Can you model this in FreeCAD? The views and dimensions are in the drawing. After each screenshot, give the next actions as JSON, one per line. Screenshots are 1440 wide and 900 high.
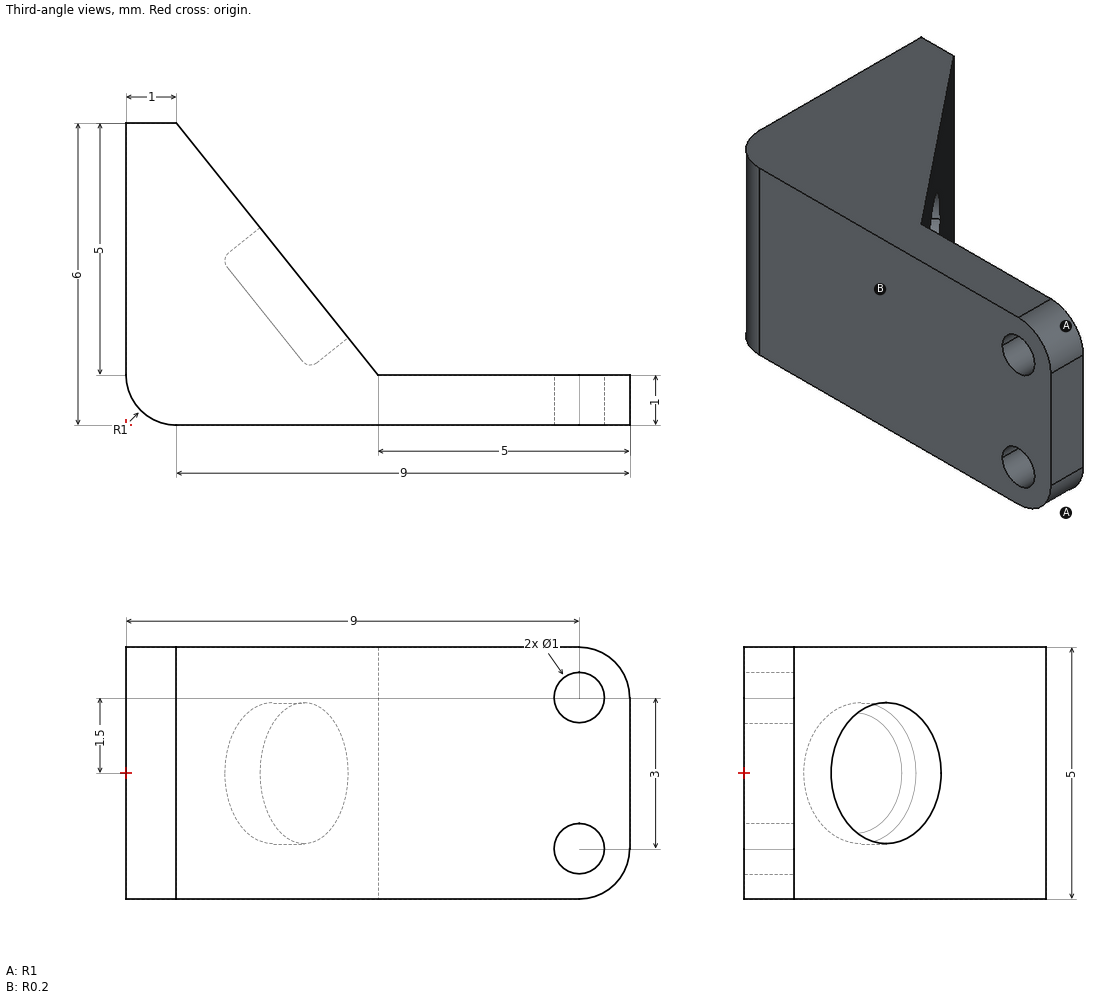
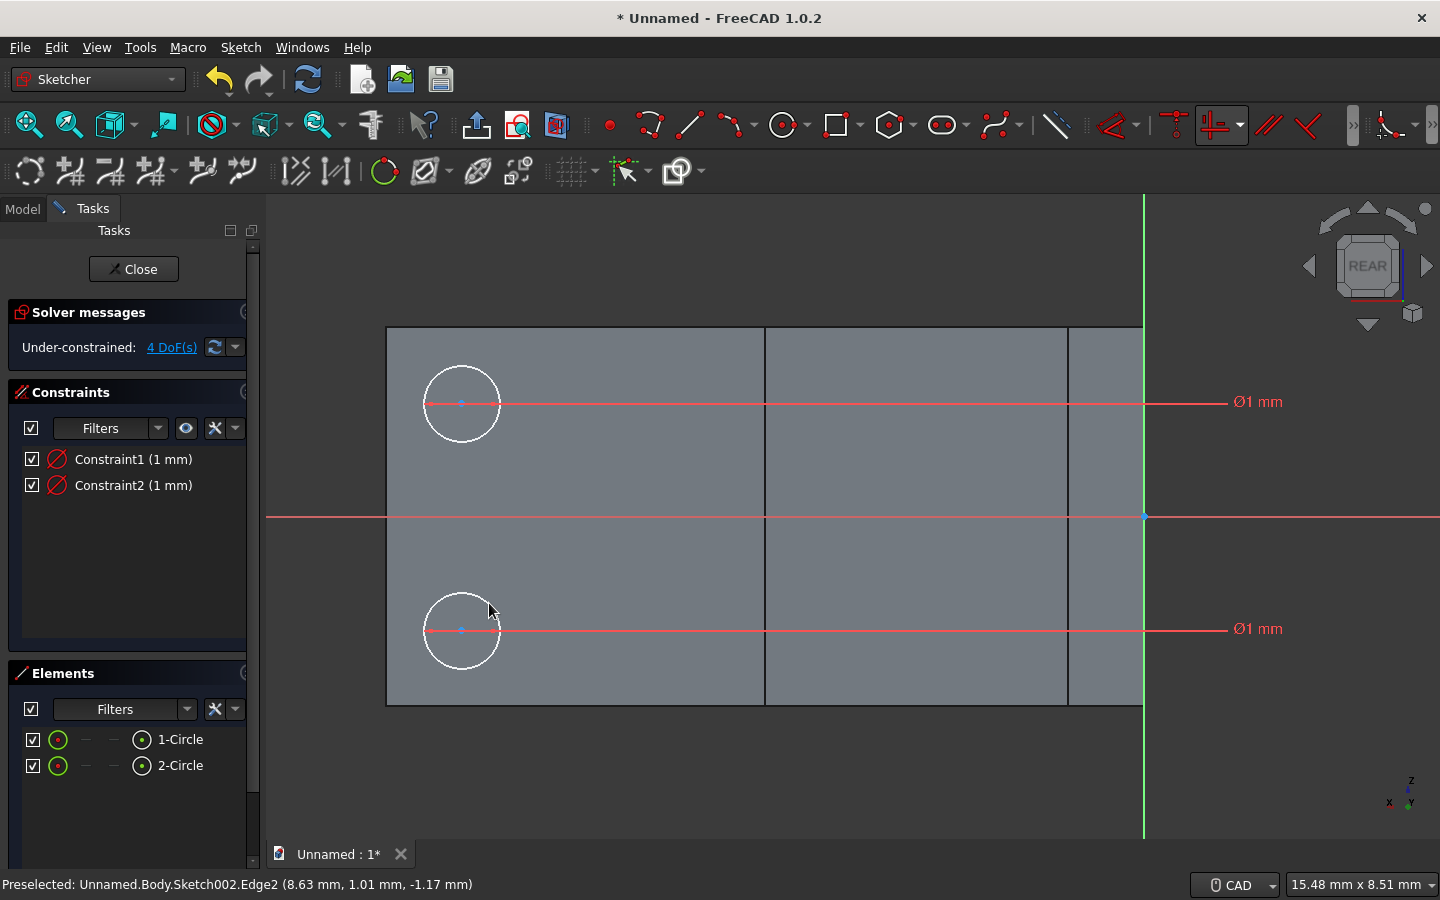
{"action": "left_click", "coordinate": [462, 404]}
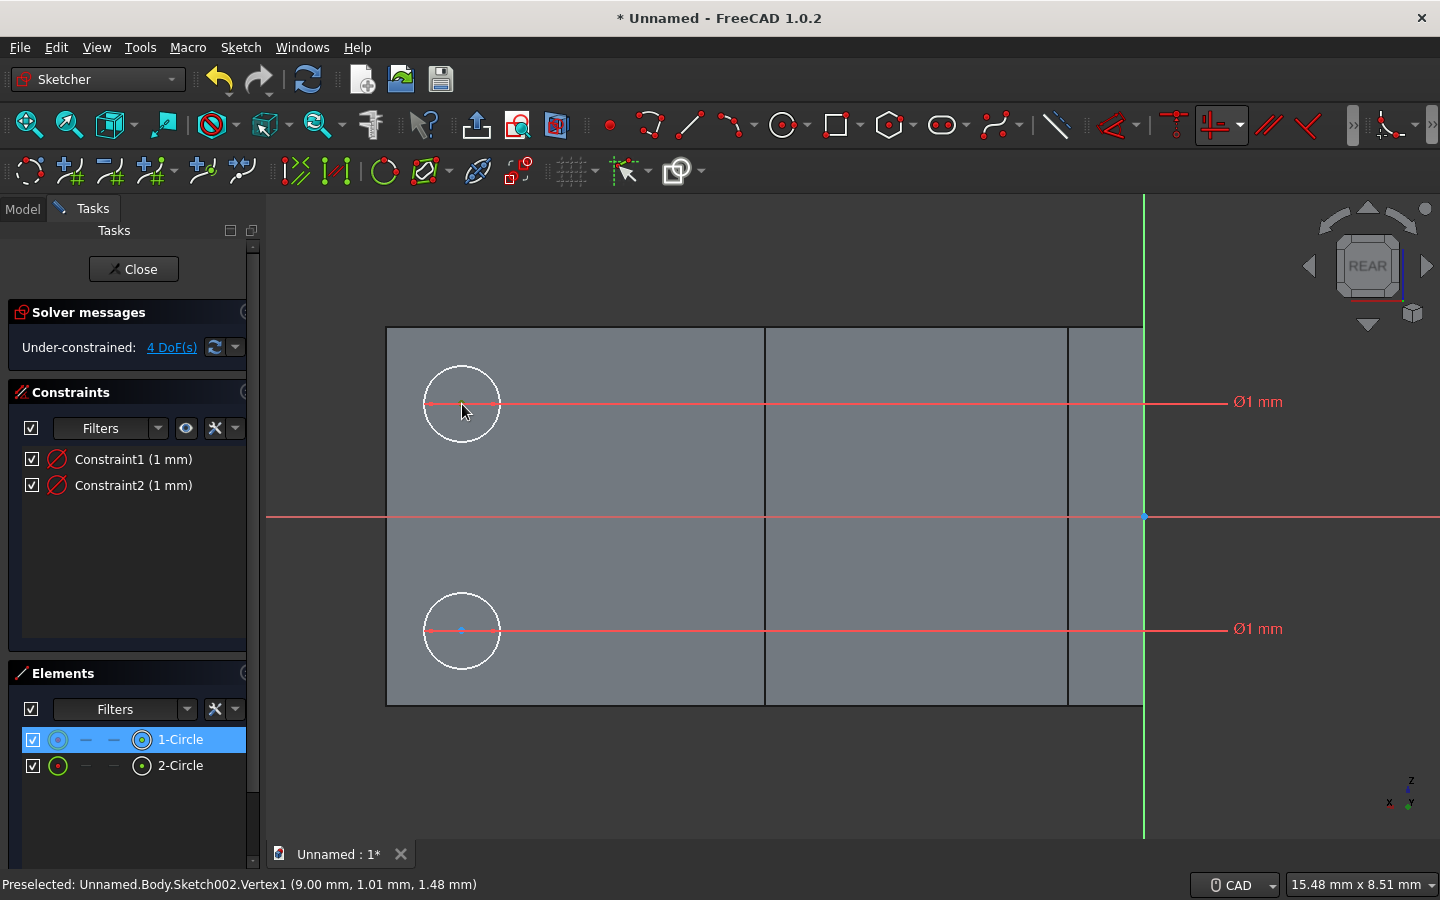
{"action": "left_click", "coordinate": [462, 631]}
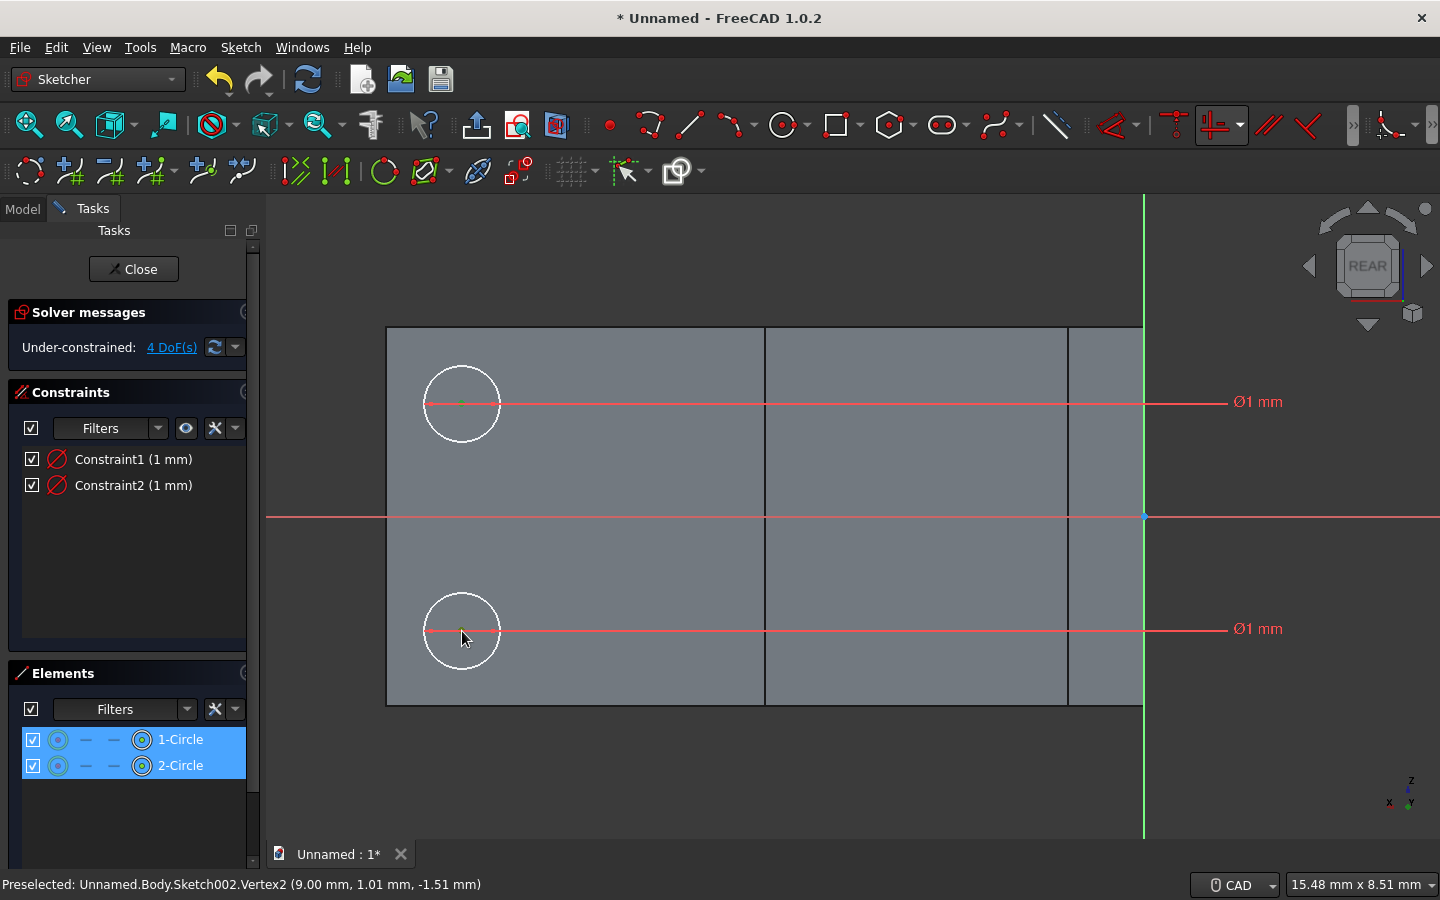
{"action": "key", "text": "v"}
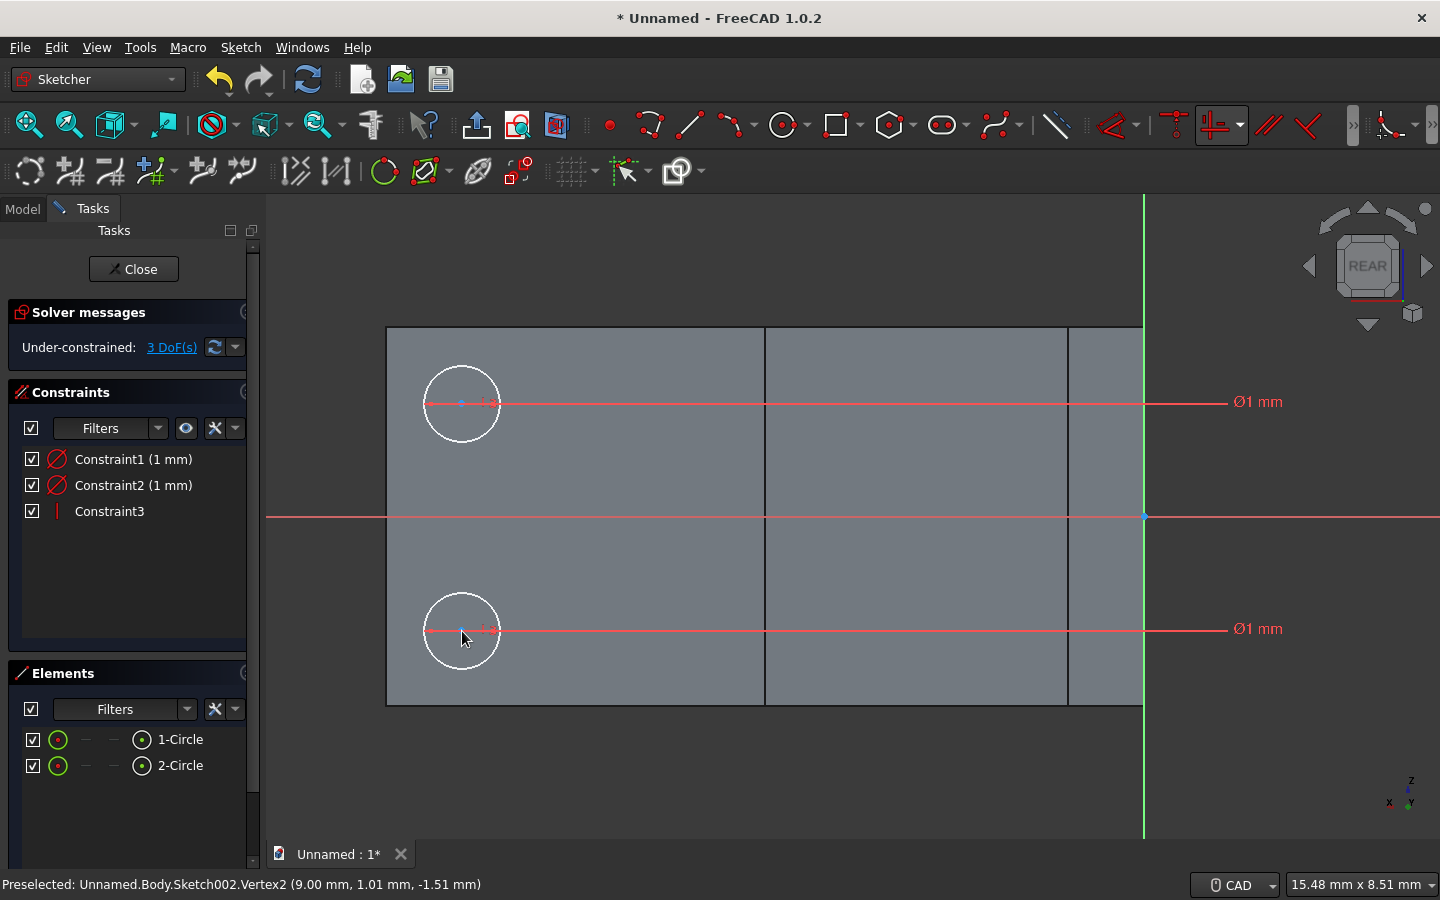
{"action": "left_click", "coordinate": [1112, 126]}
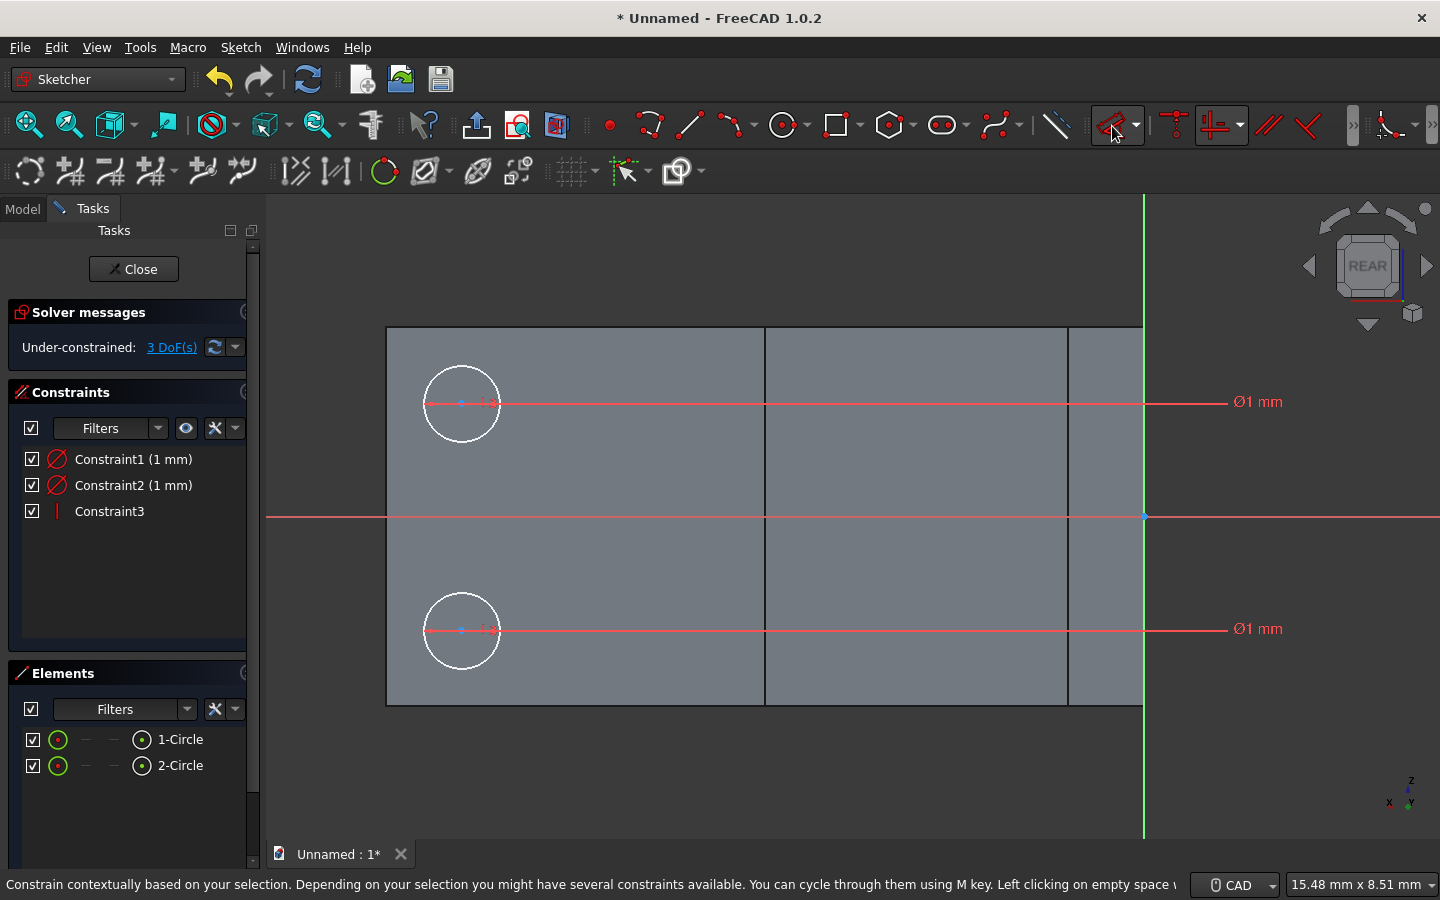
{"action": "left_click", "coordinate": [462, 404]}
{"action": "left_click", "coordinate": [803, 370]}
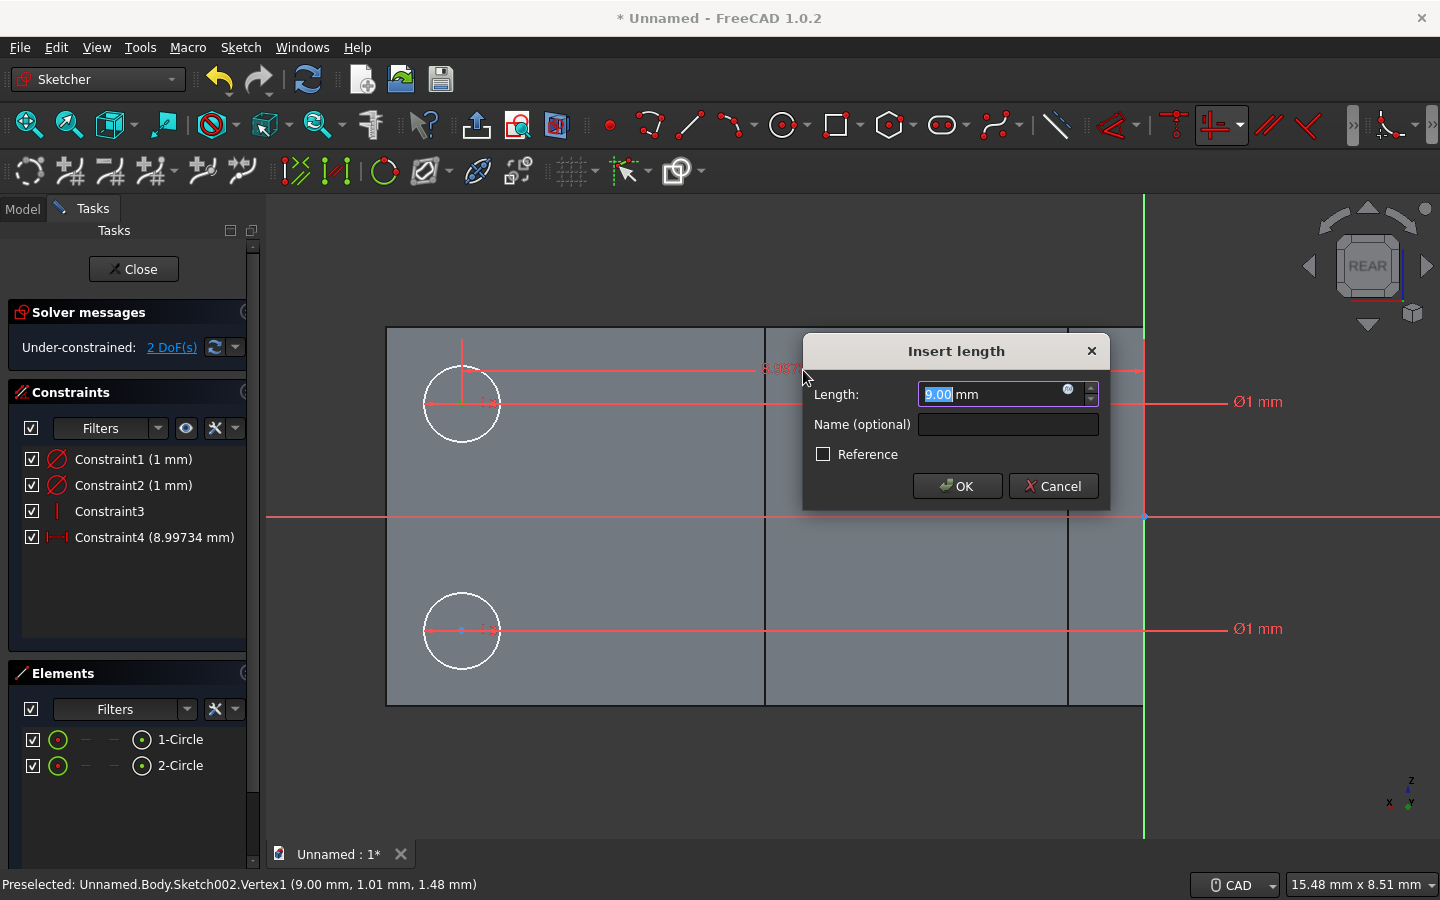
{"action": "type", "text": "9"}
{"action": "key", "text": "Return"}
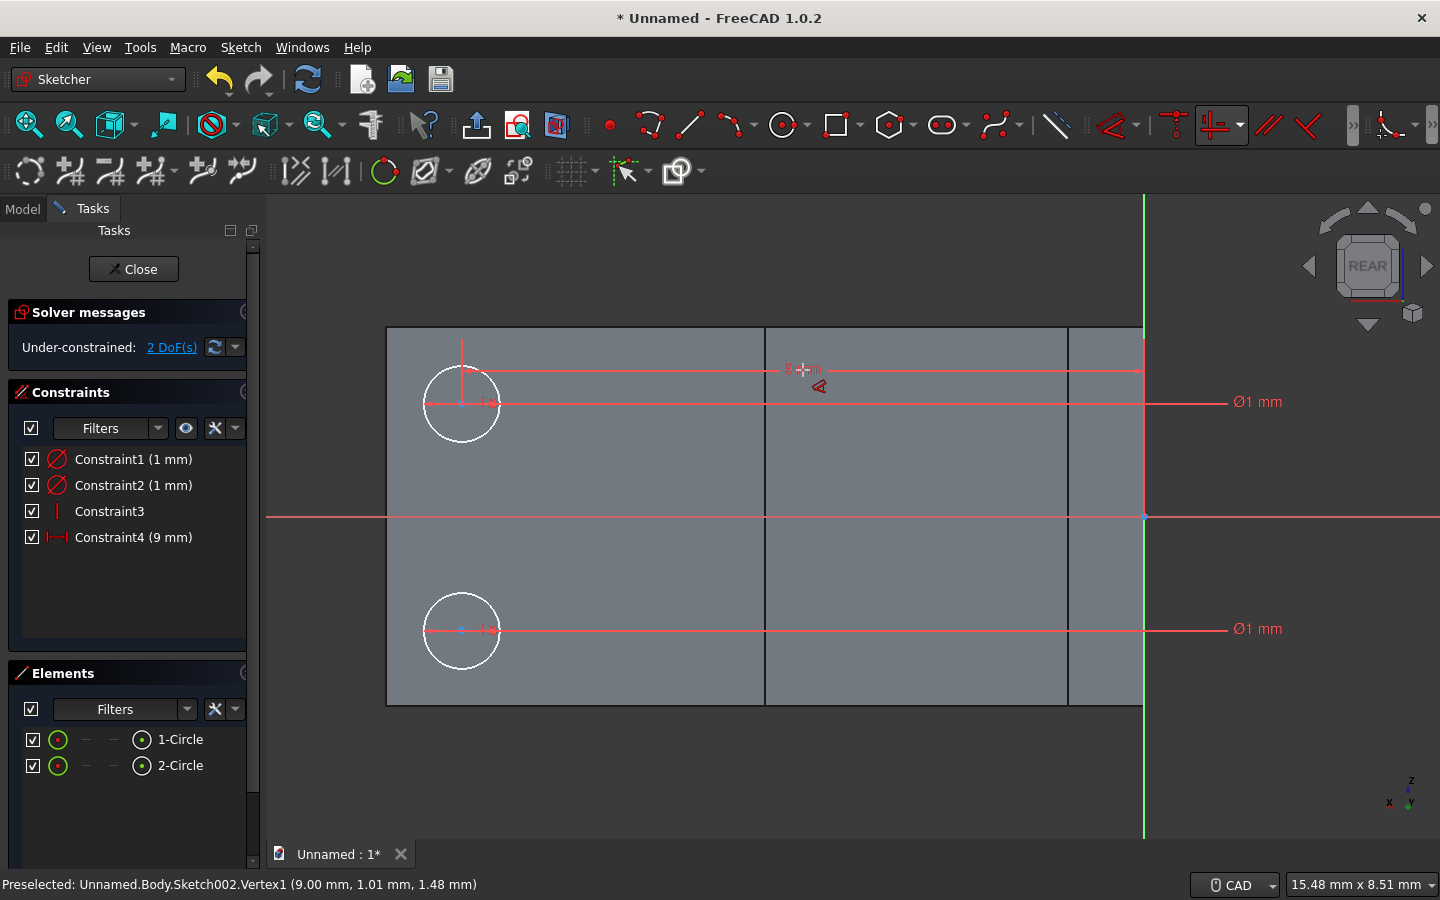
{"action": "left_click", "coordinate": [462, 404]}